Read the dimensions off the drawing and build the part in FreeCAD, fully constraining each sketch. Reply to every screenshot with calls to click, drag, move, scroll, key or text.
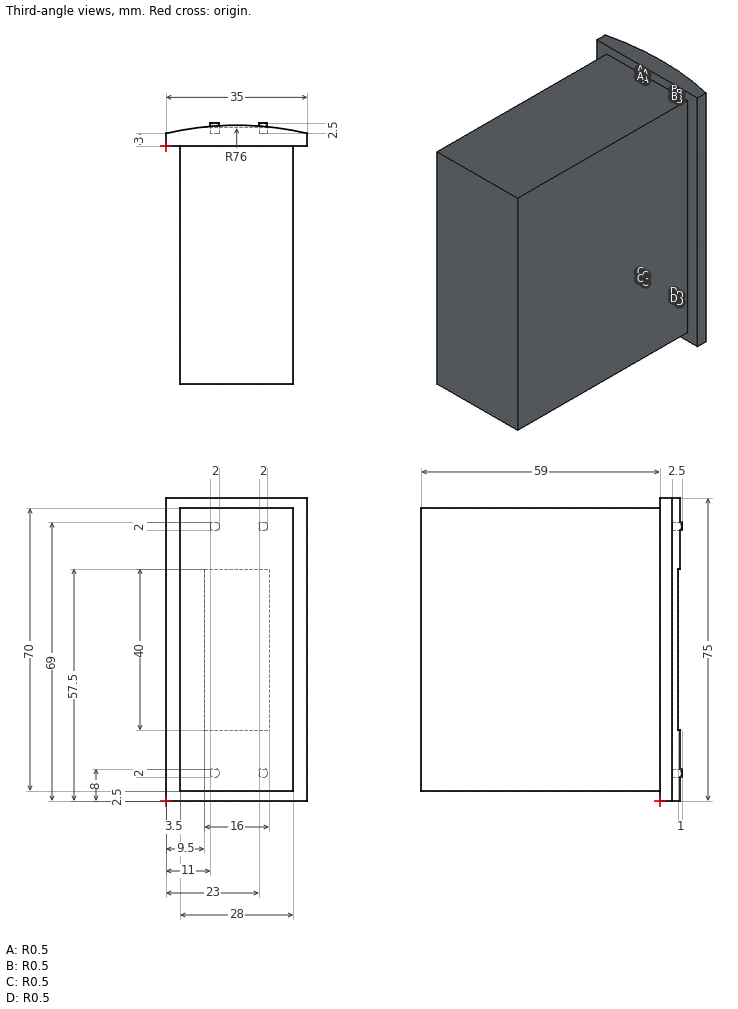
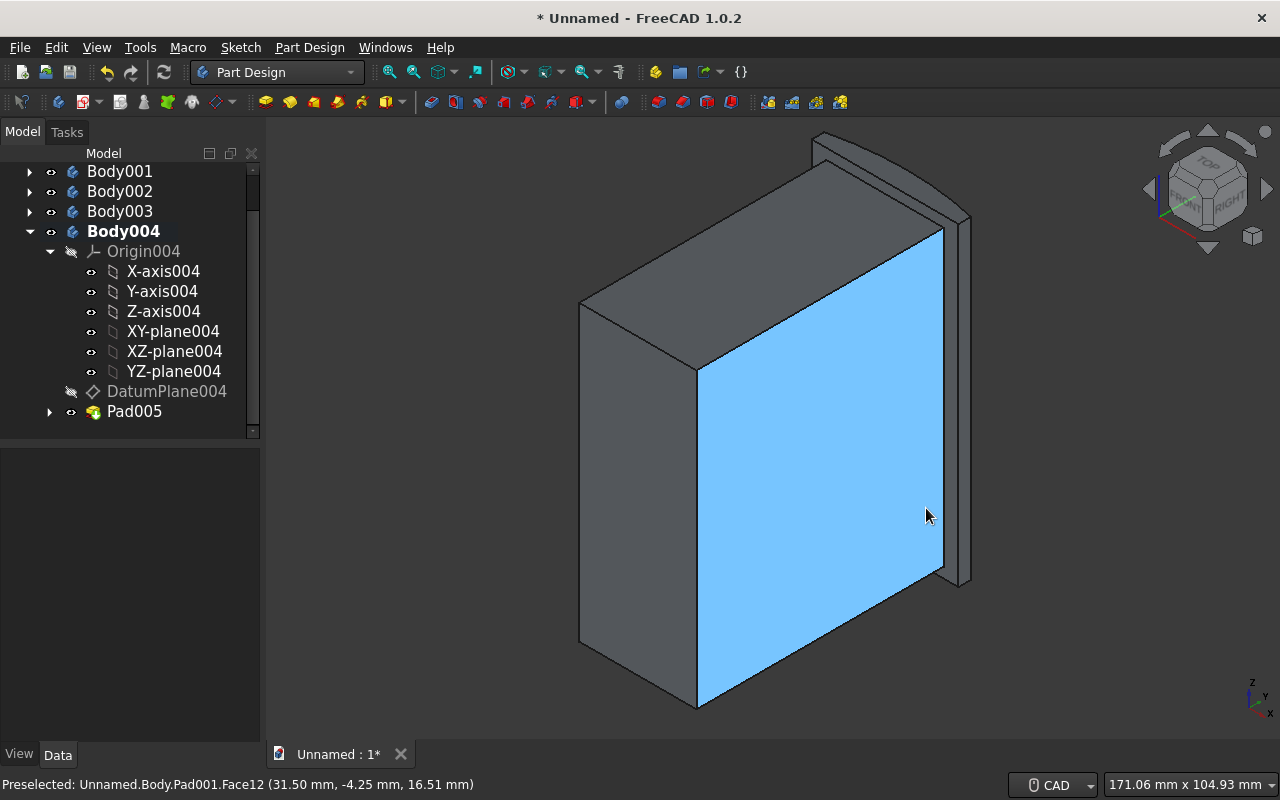
key(2)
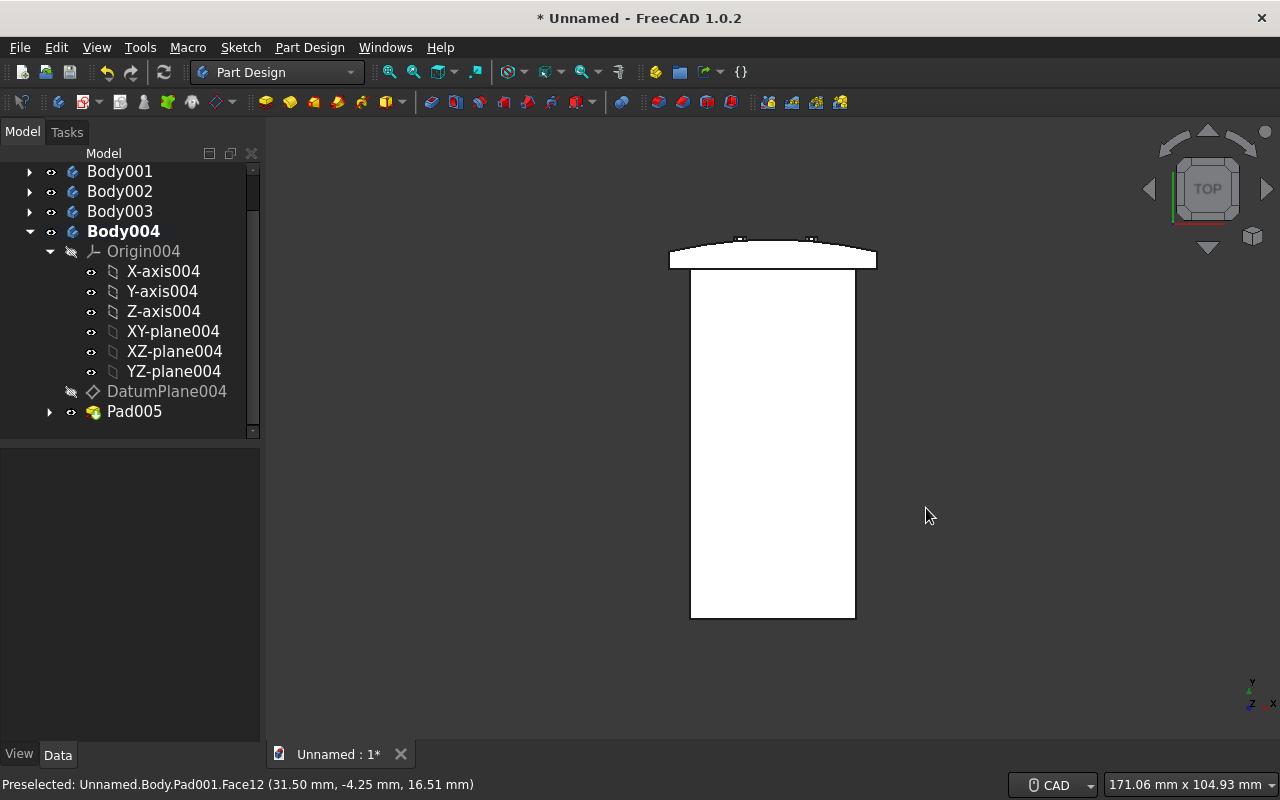
click(390, 72)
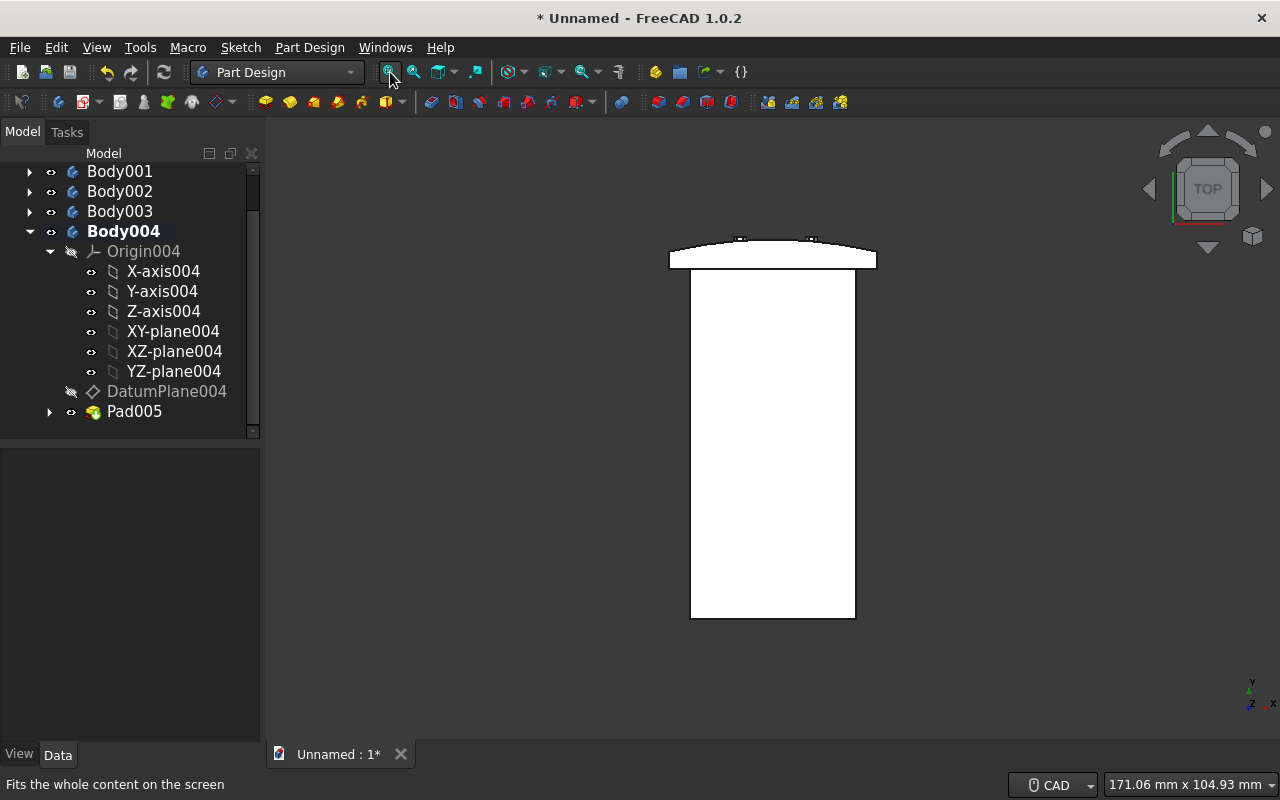
scroll(806, 243, up, 5)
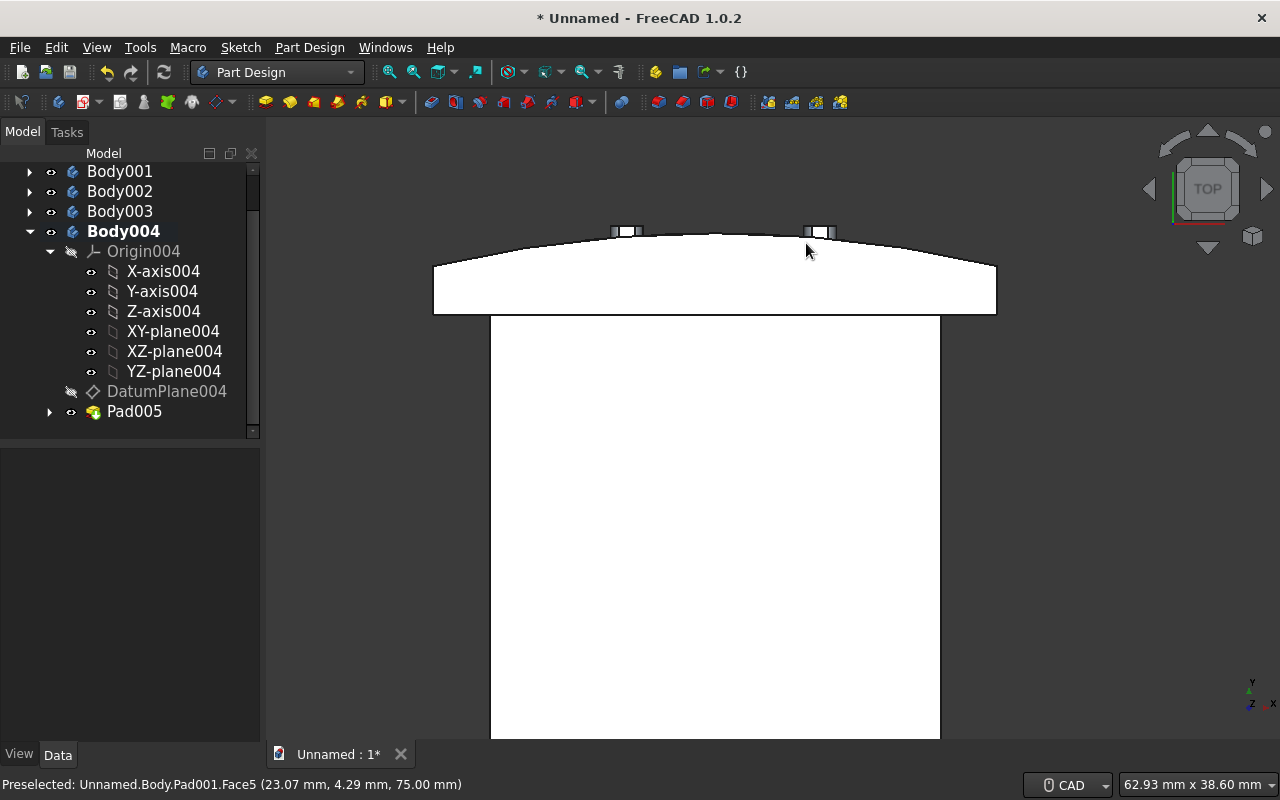
key(v)
key(f)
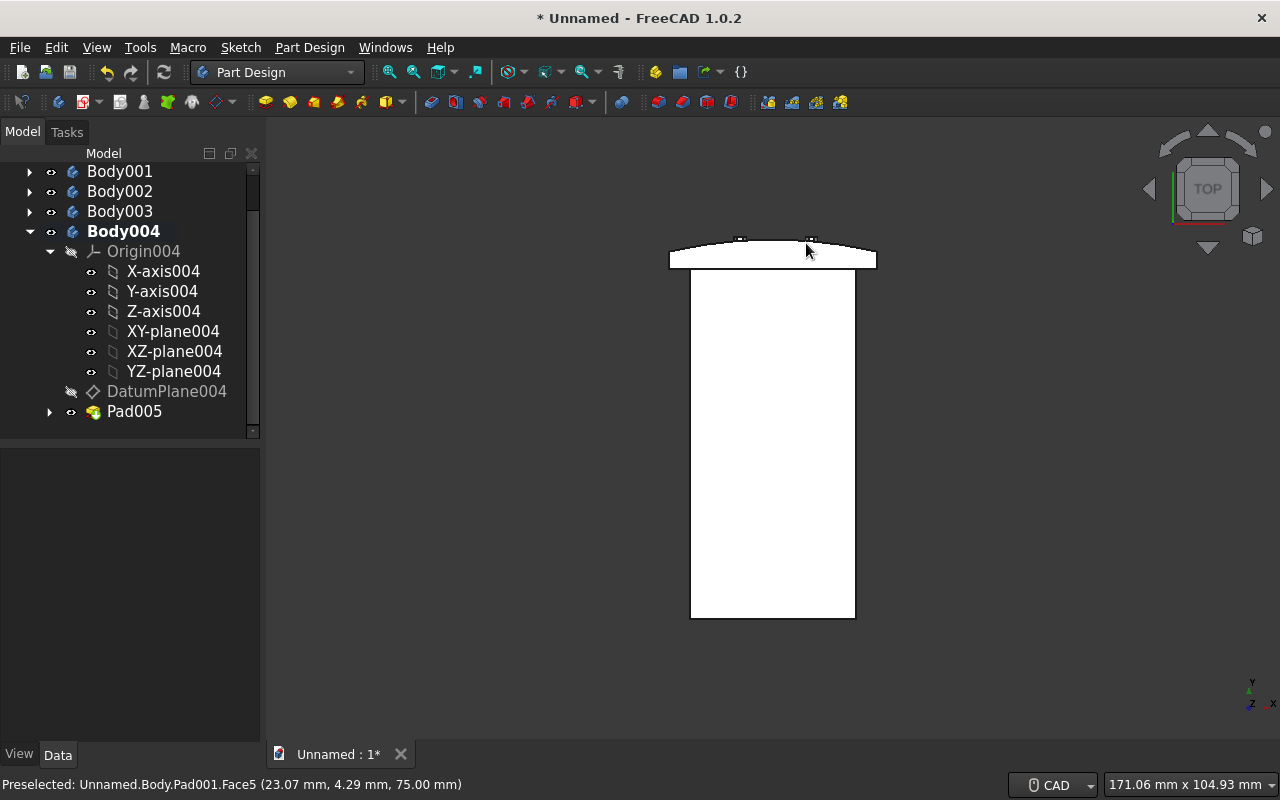
key(0)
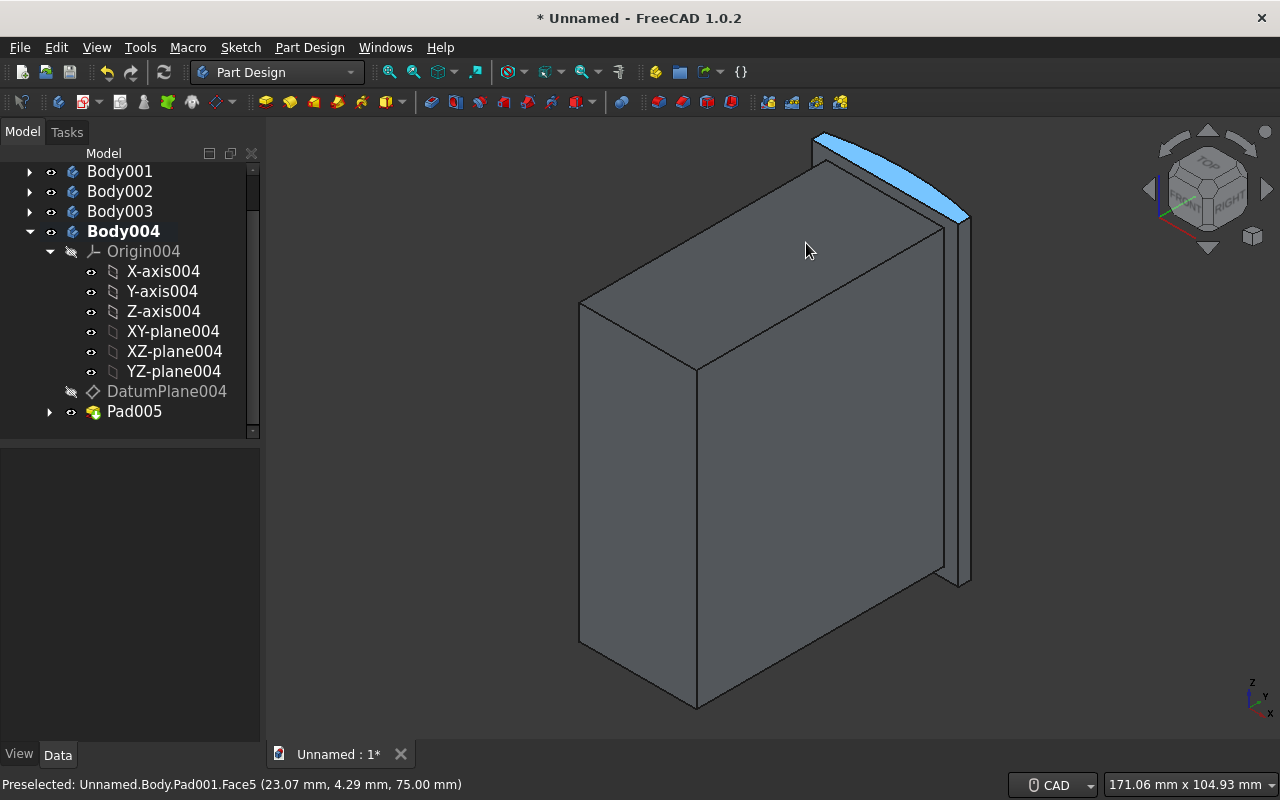
key(v)
key(f)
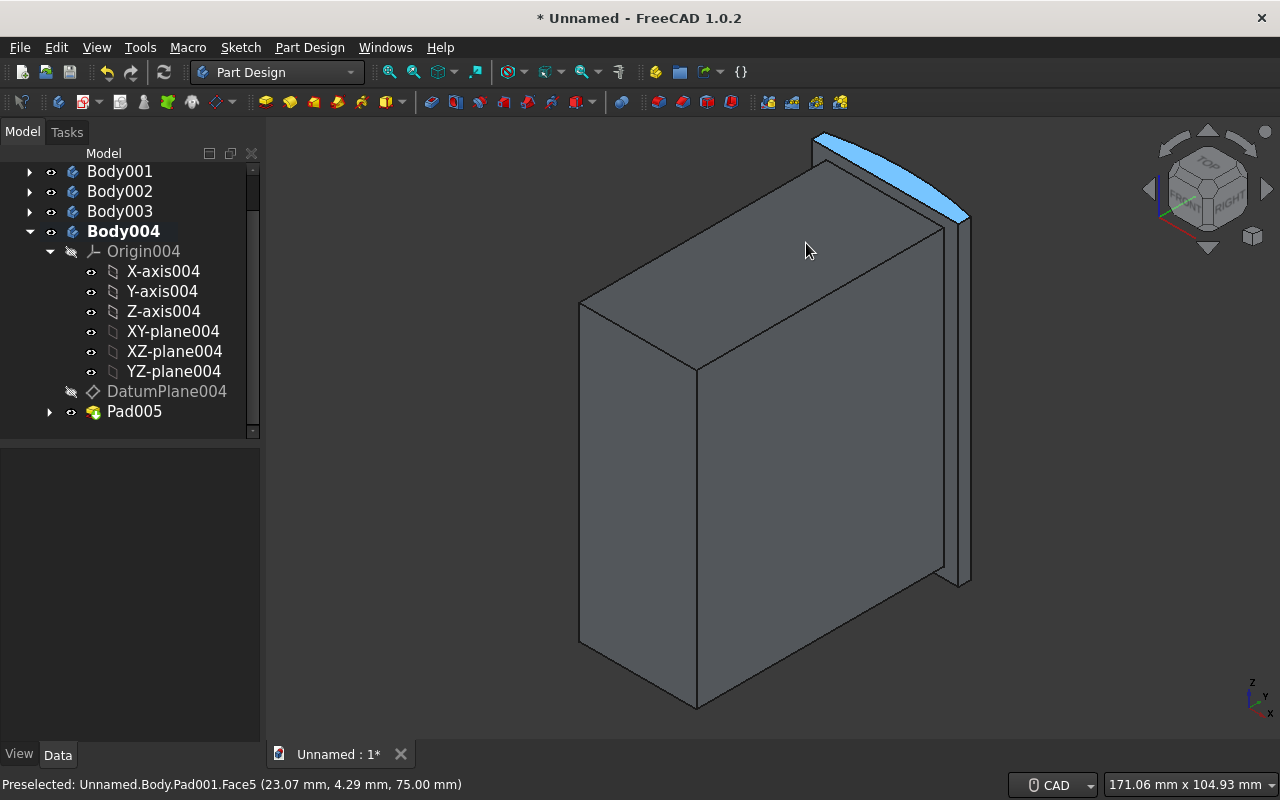
scroll(926, 508, up, 5)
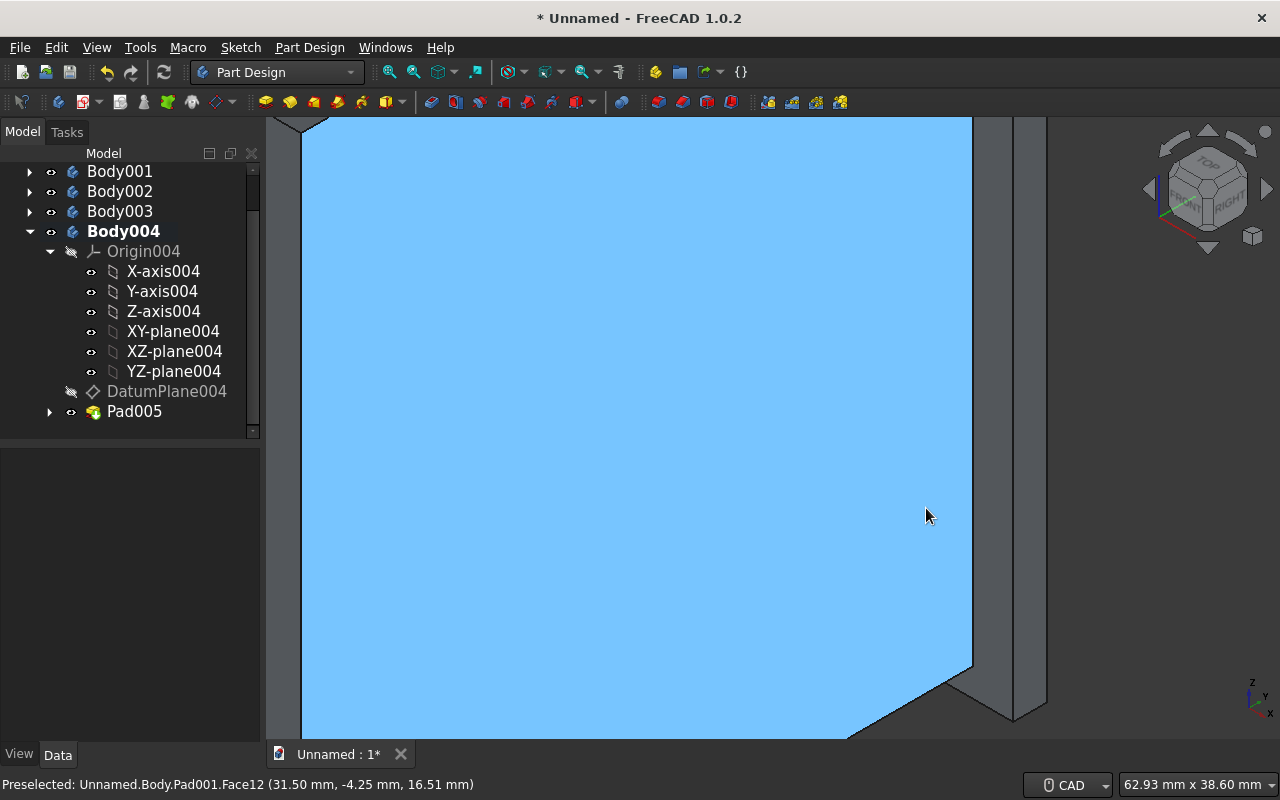
key(v)
key(f)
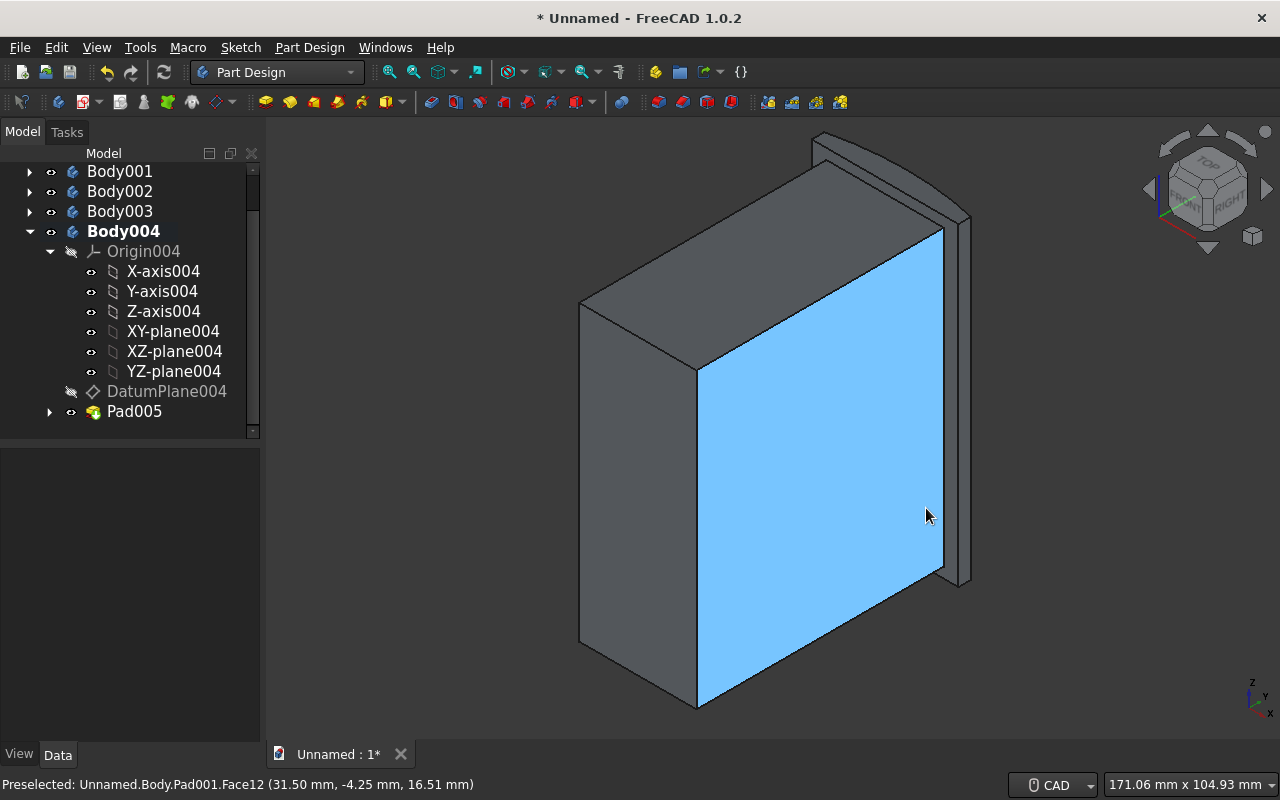
key(1)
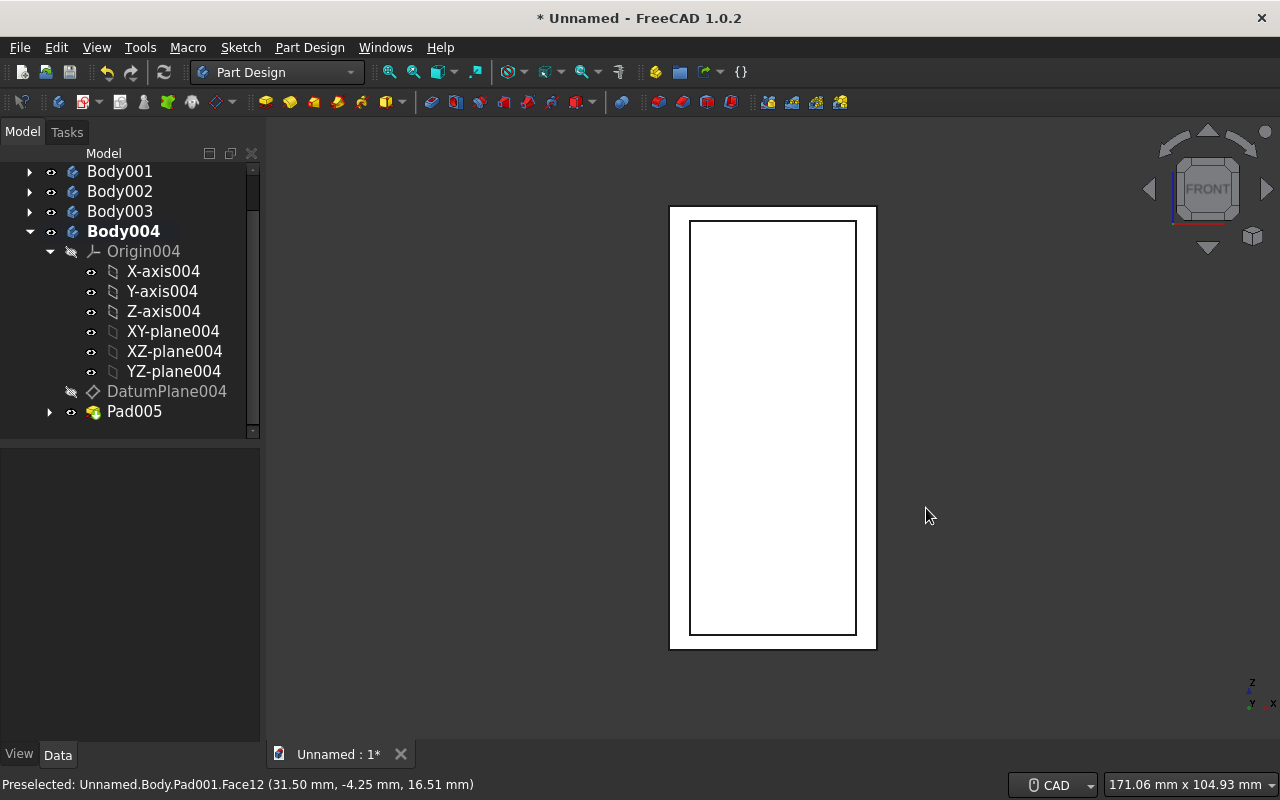
key(v)
key(f)